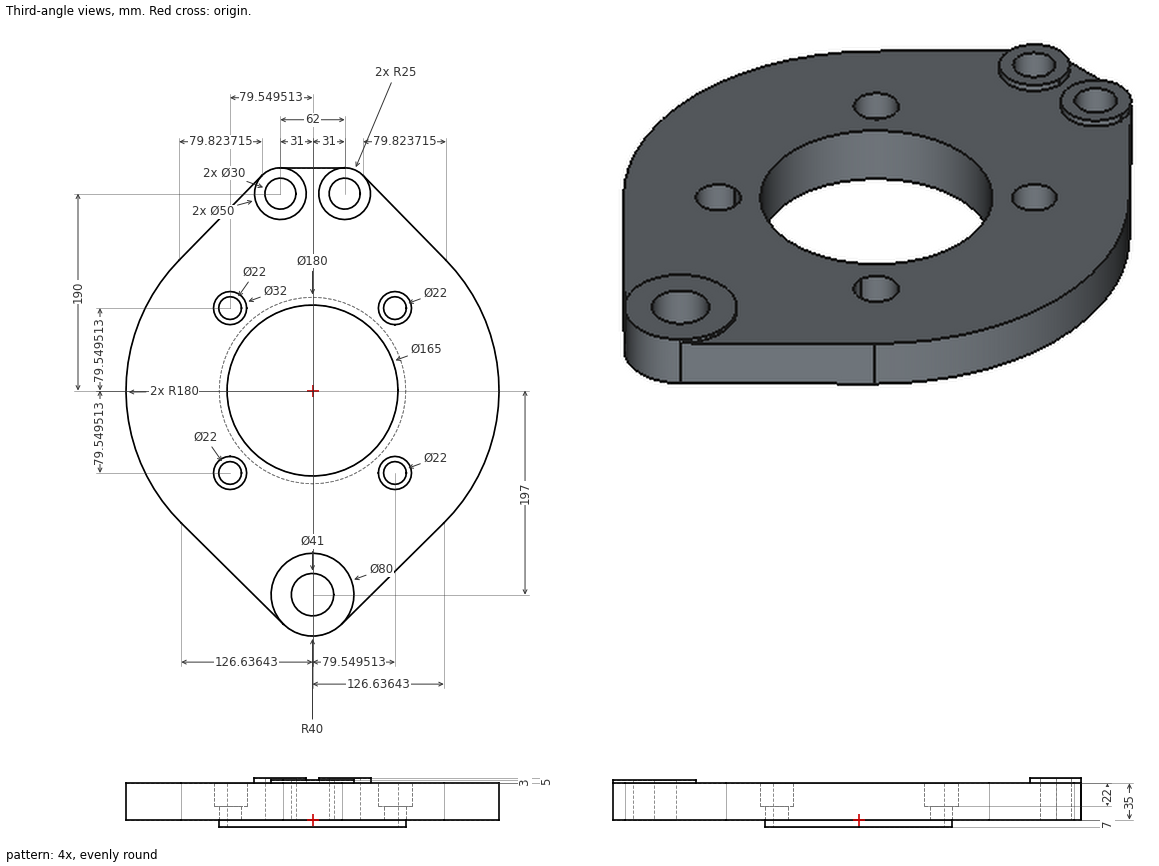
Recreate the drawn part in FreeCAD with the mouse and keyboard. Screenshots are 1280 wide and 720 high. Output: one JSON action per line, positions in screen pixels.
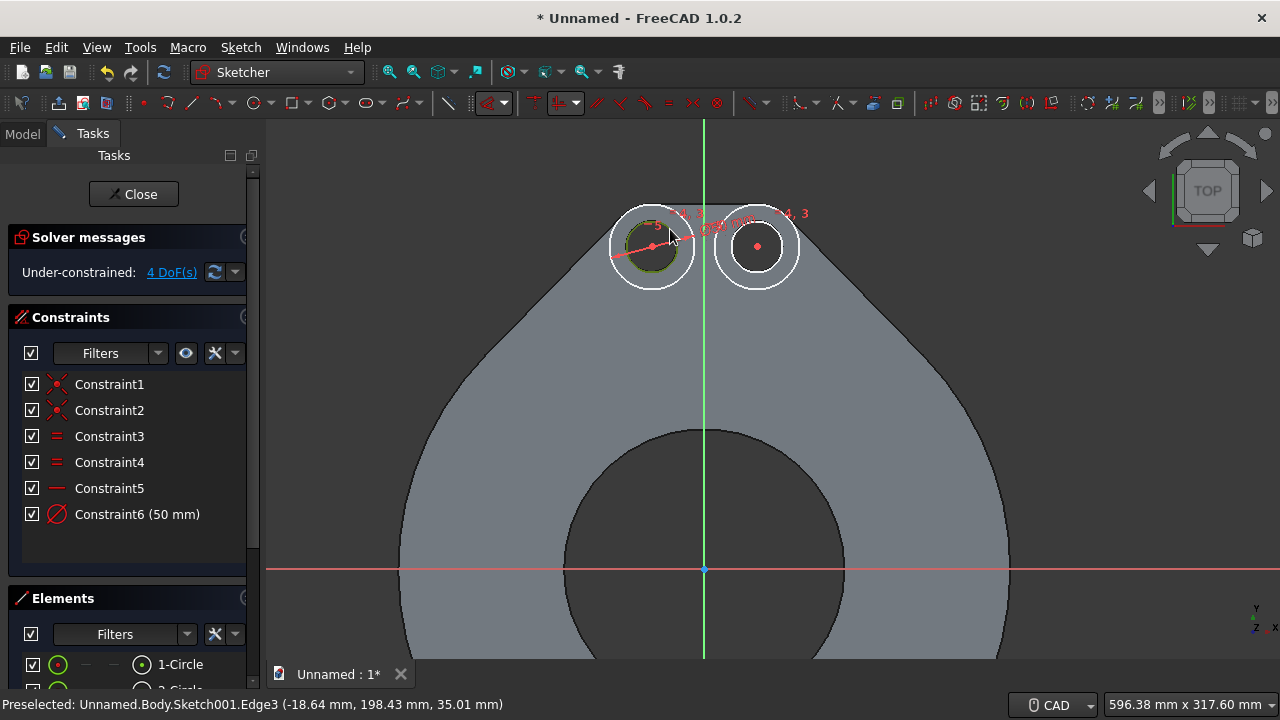
{"action": "key", "text": "k o"}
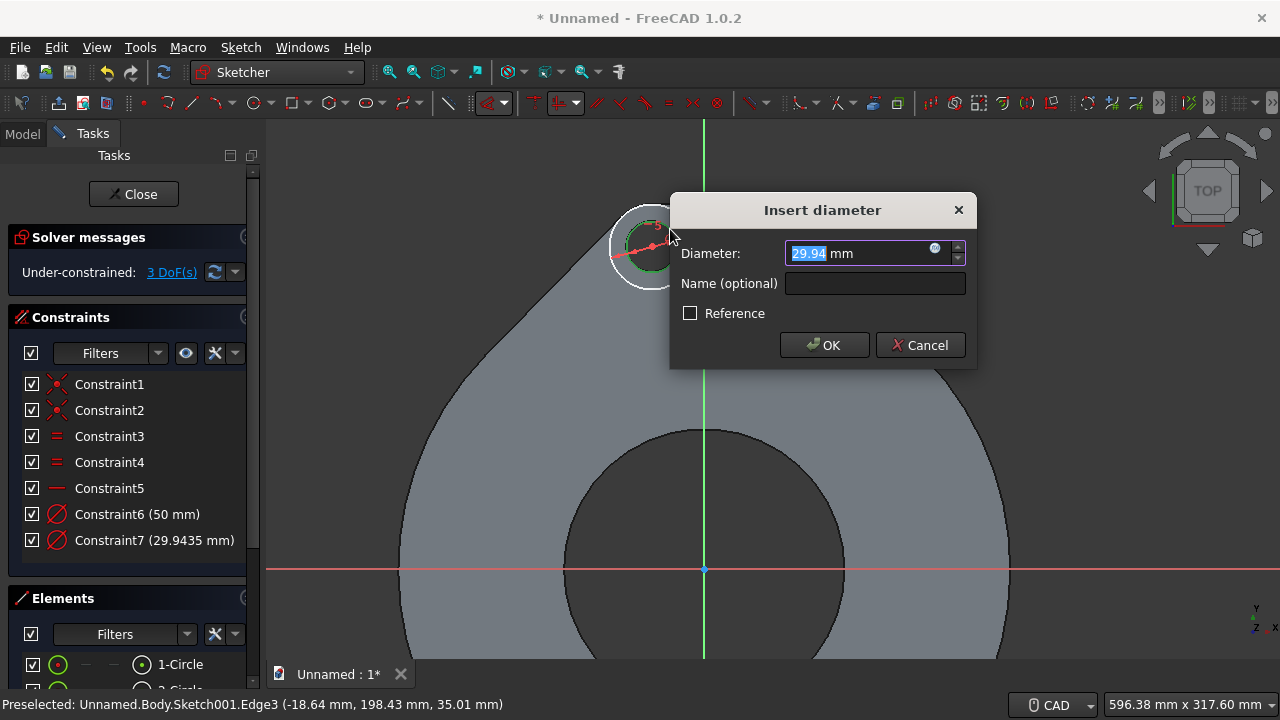
{"action": "type", "text": "30"}
{"action": "key", "text": "Return"}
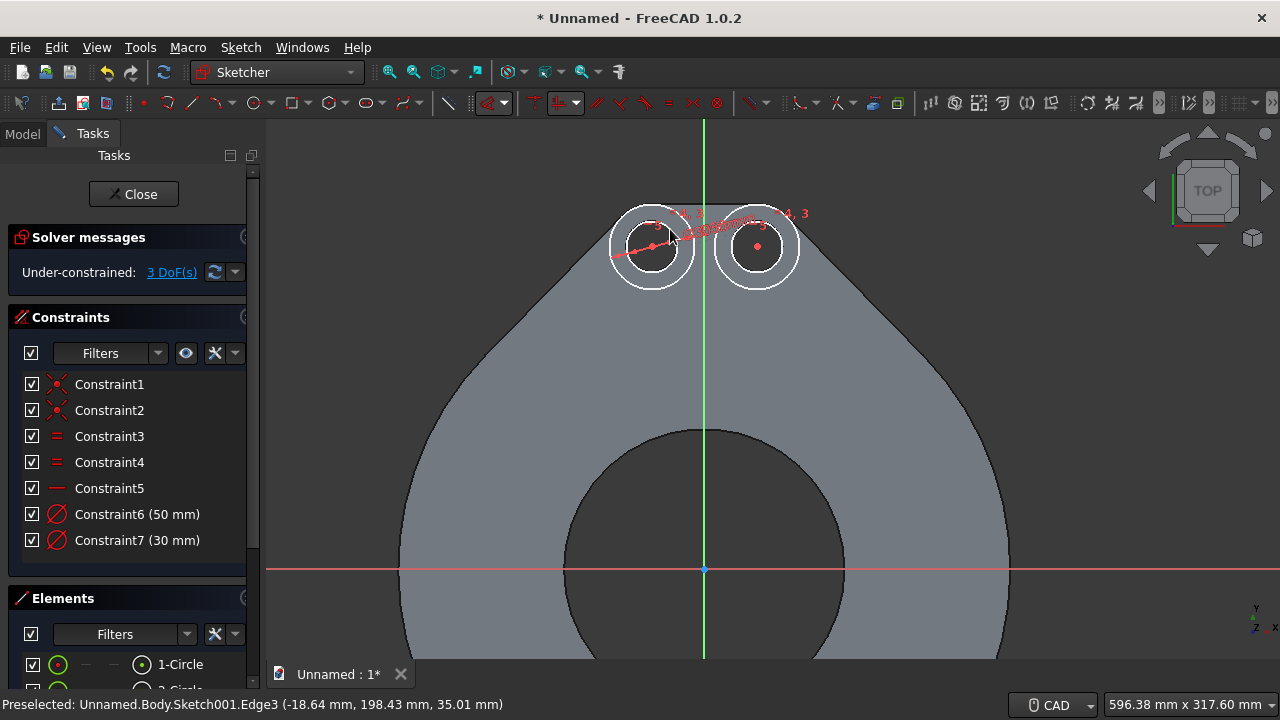
{"action": "left_click", "coordinate": [652, 247]}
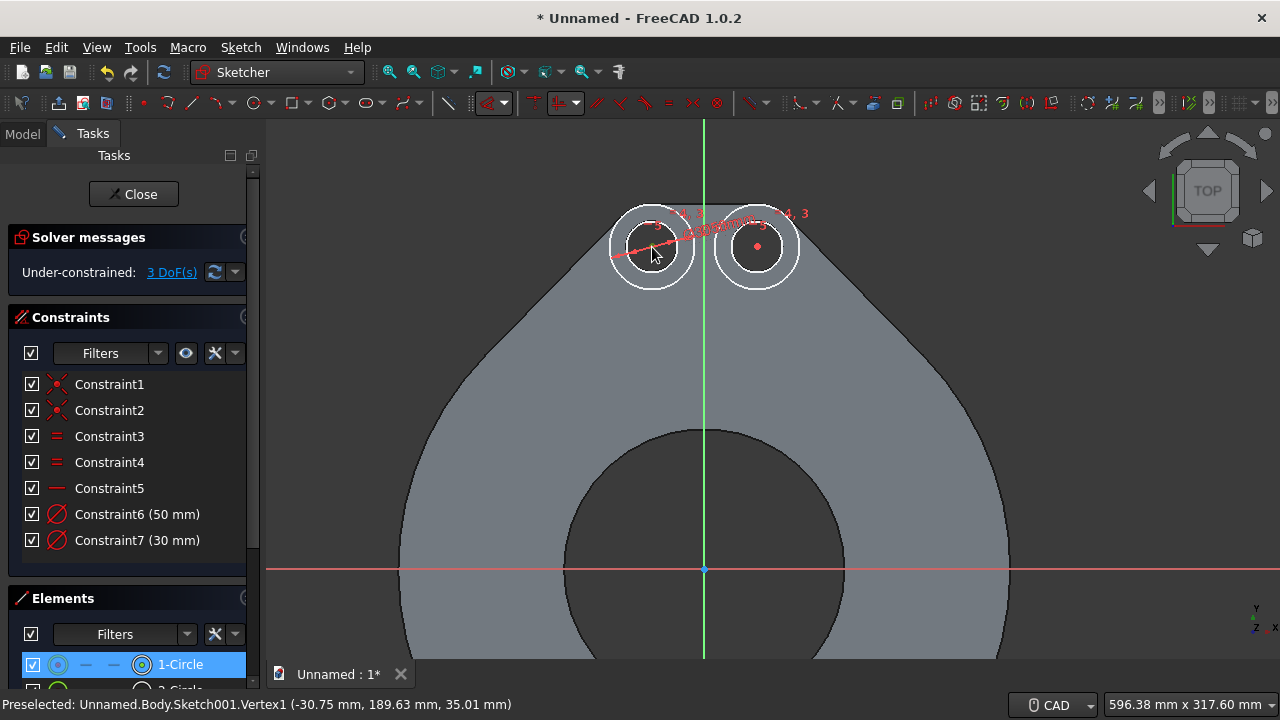
{"action": "key", "text": "l"}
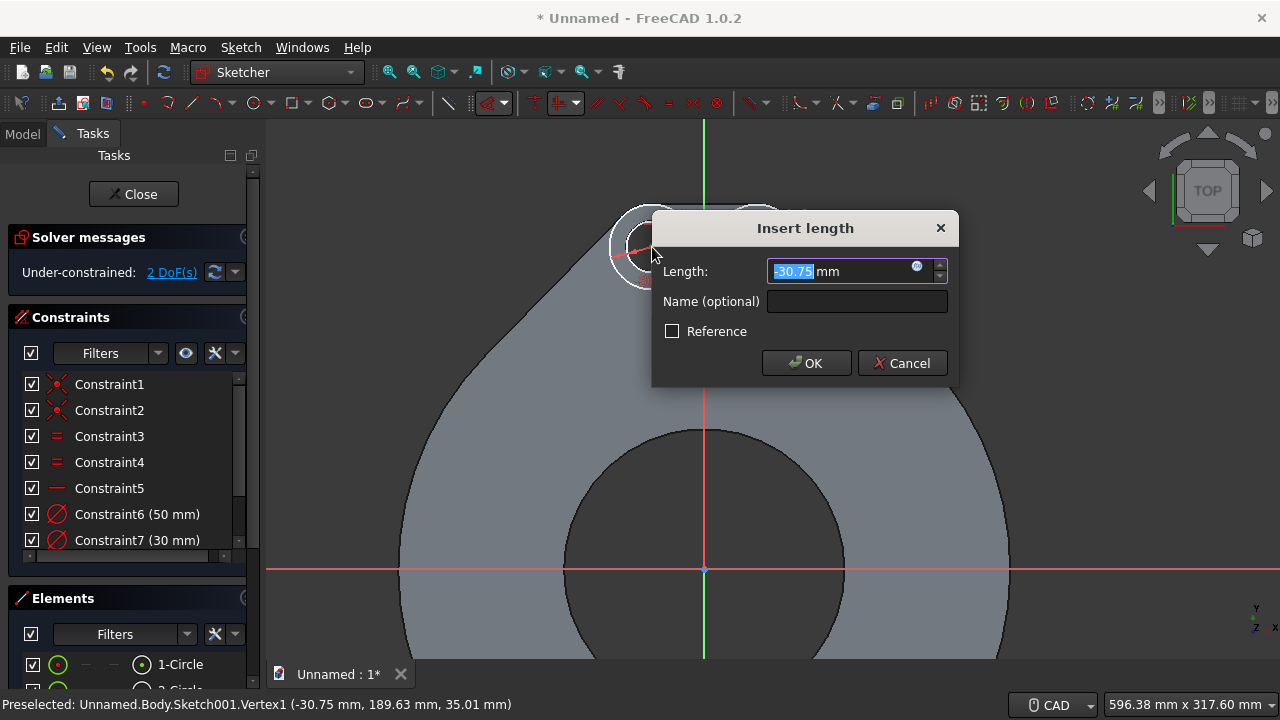
{"action": "type", "text": "-31"}
{"action": "key", "text": "Return"}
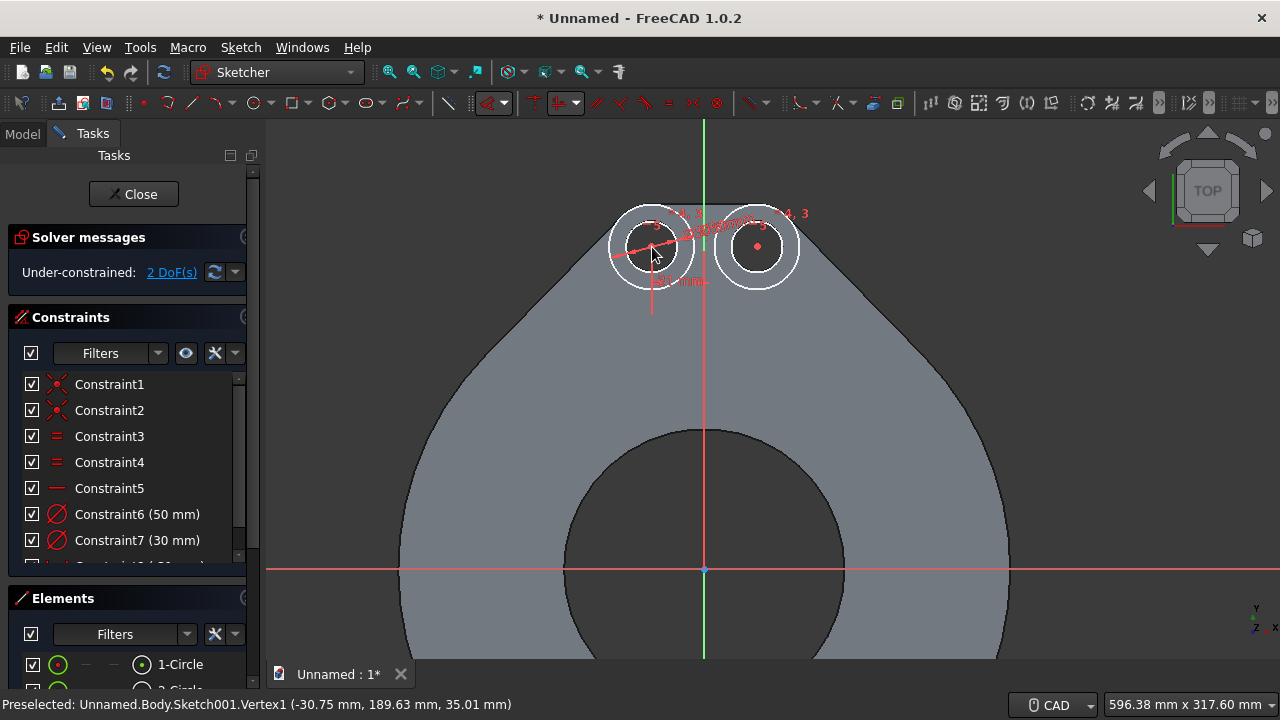
{"action": "left_click", "coordinate": [757, 247]}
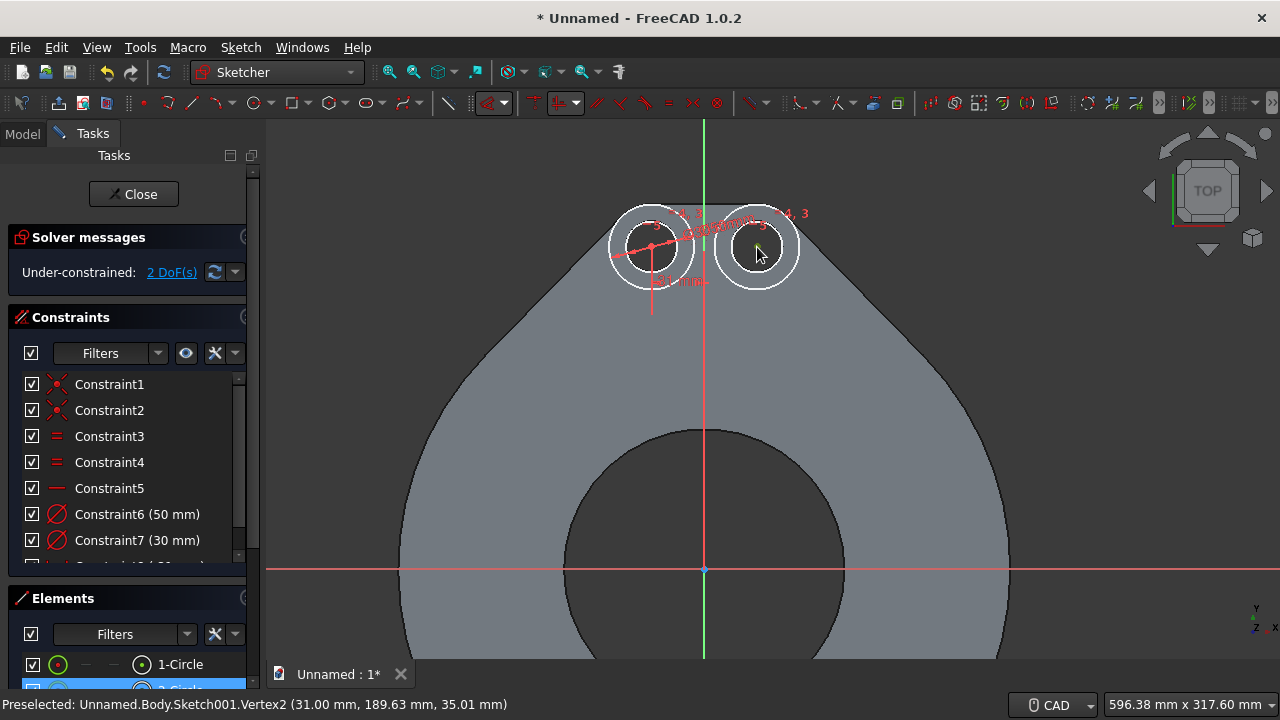
{"action": "key", "text": "l"}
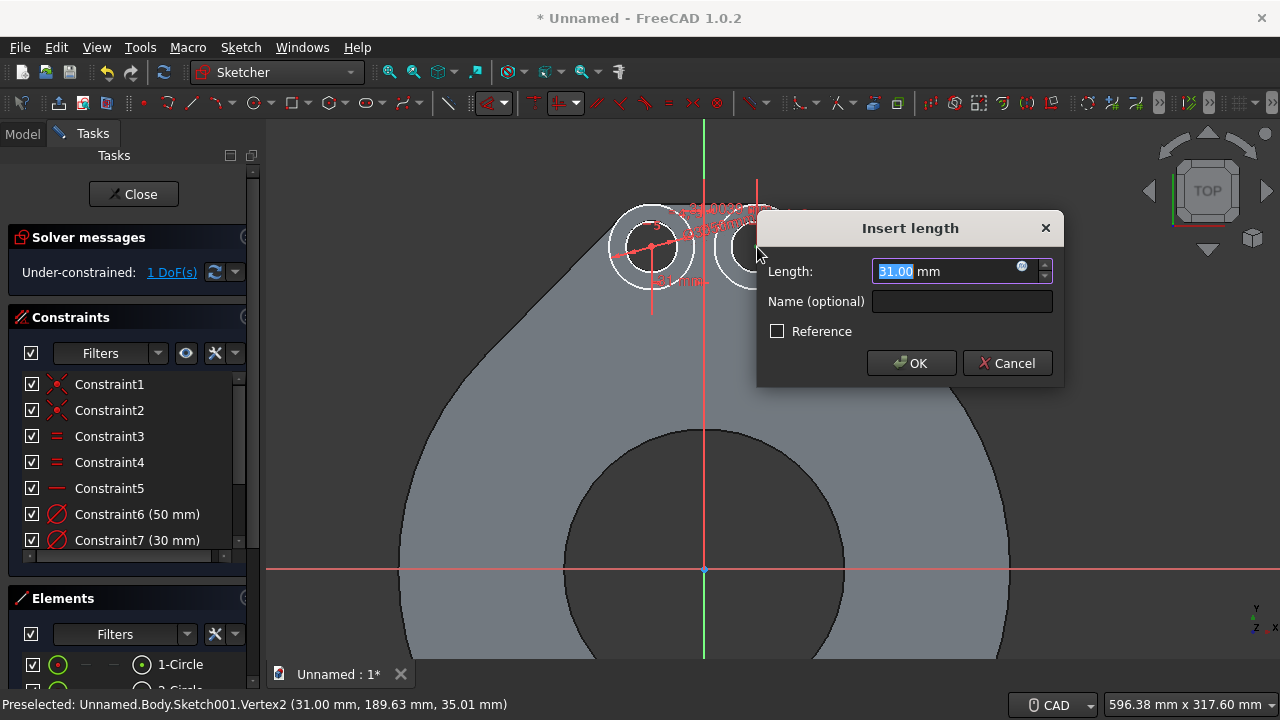
{"action": "type", "text": "31"}
{"action": "key", "text": "Return"}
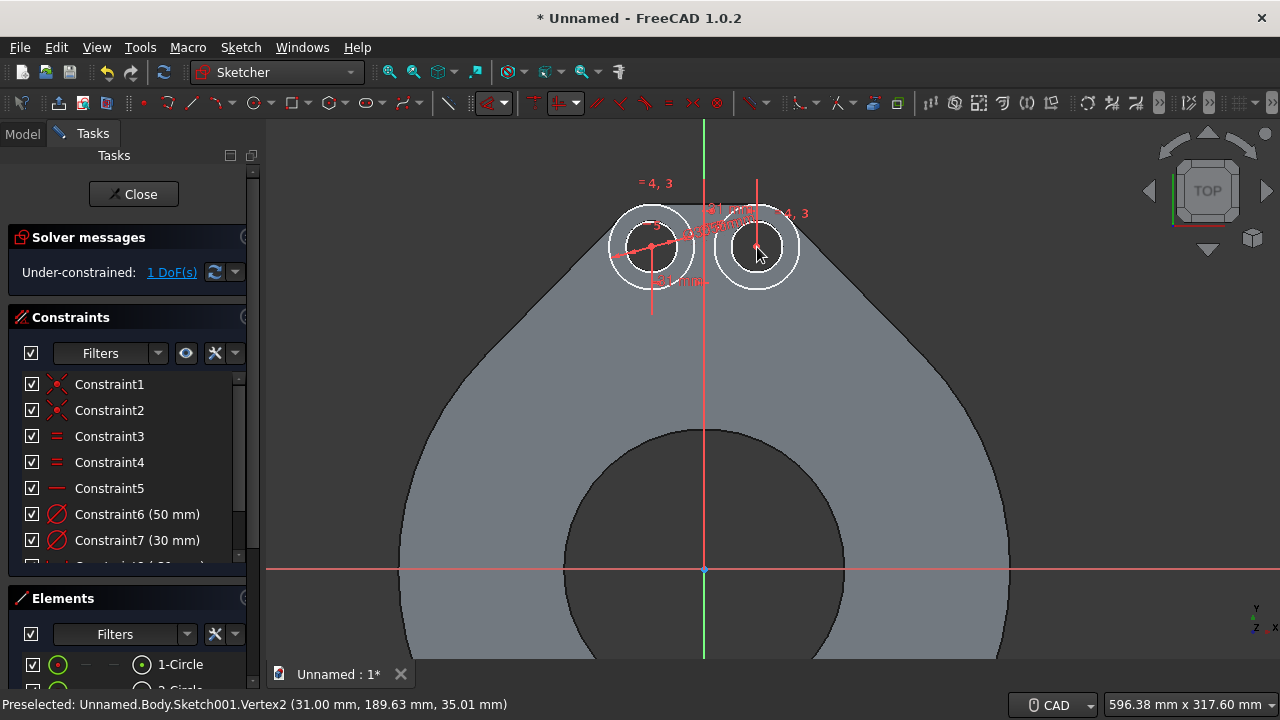
{"action": "left_click", "coordinate": [652, 247]}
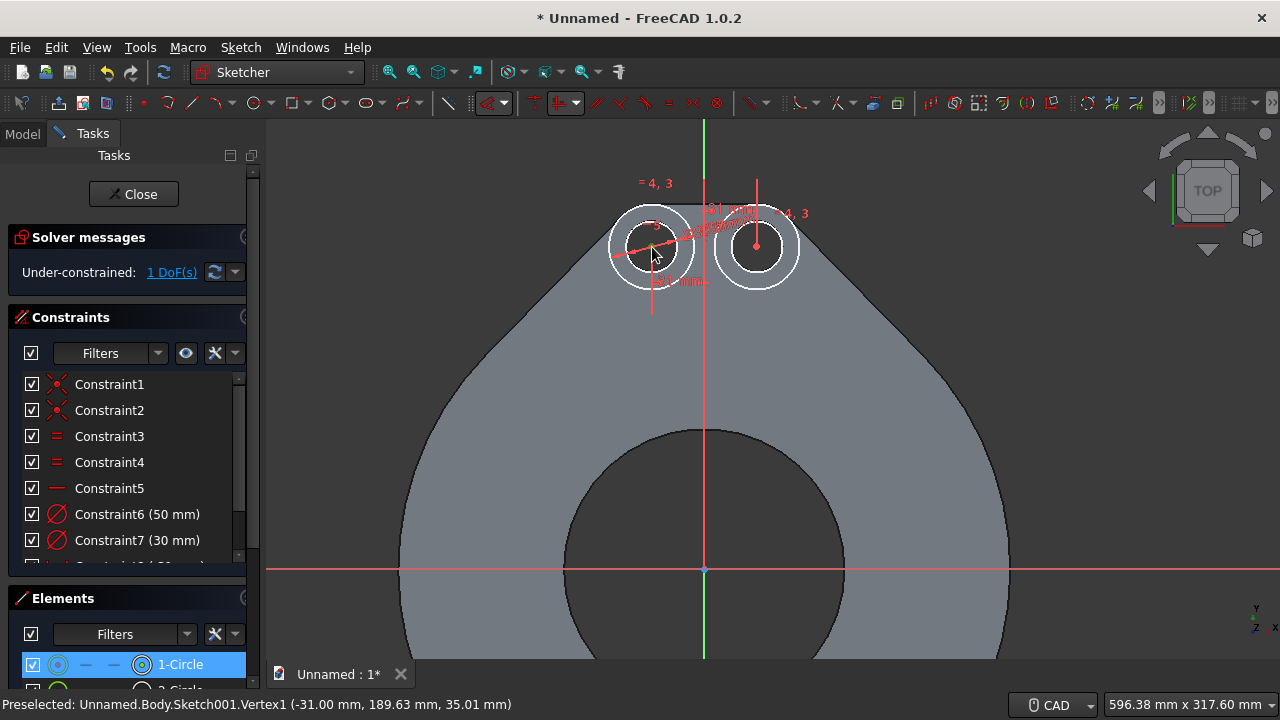
{"action": "key", "text": "i"}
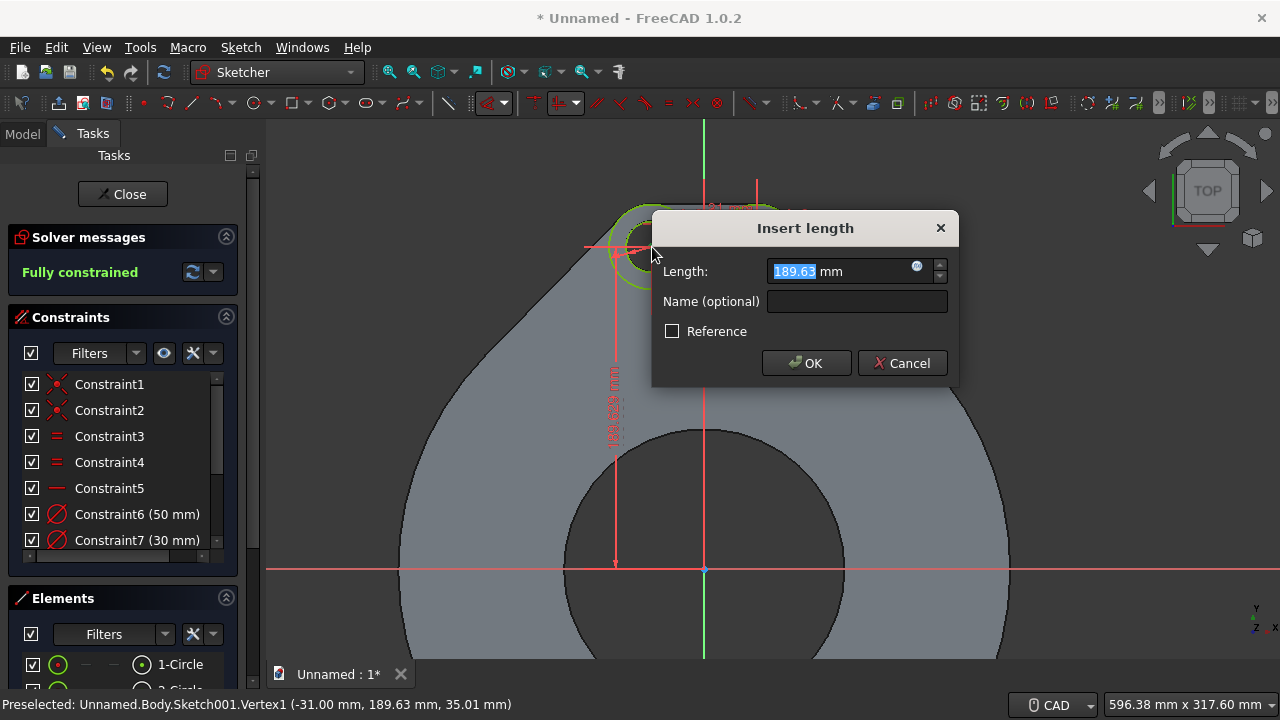
{"action": "type", "text": "190"}
{"action": "key", "text": "Return"}